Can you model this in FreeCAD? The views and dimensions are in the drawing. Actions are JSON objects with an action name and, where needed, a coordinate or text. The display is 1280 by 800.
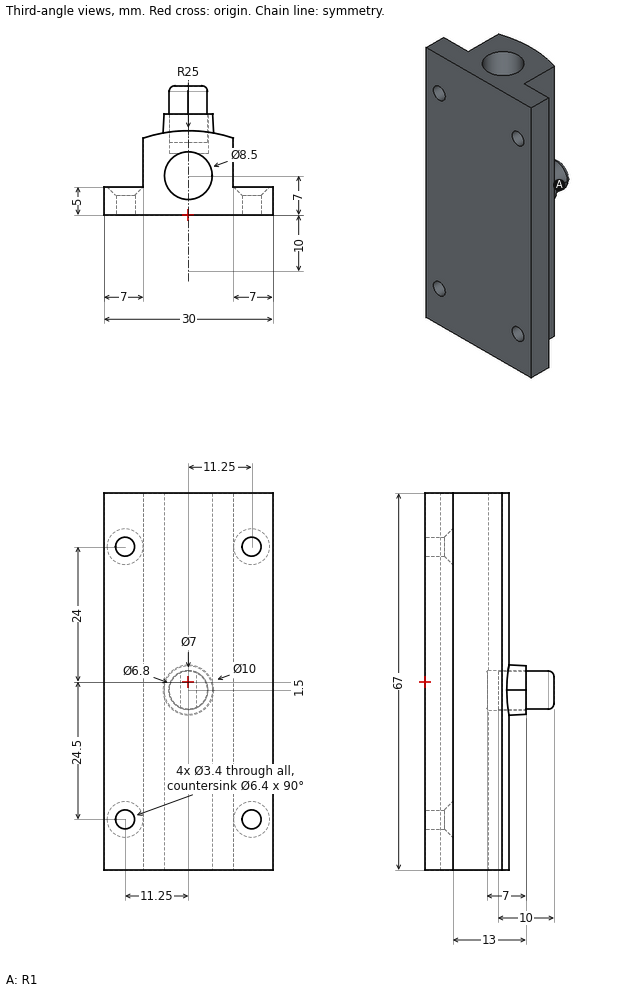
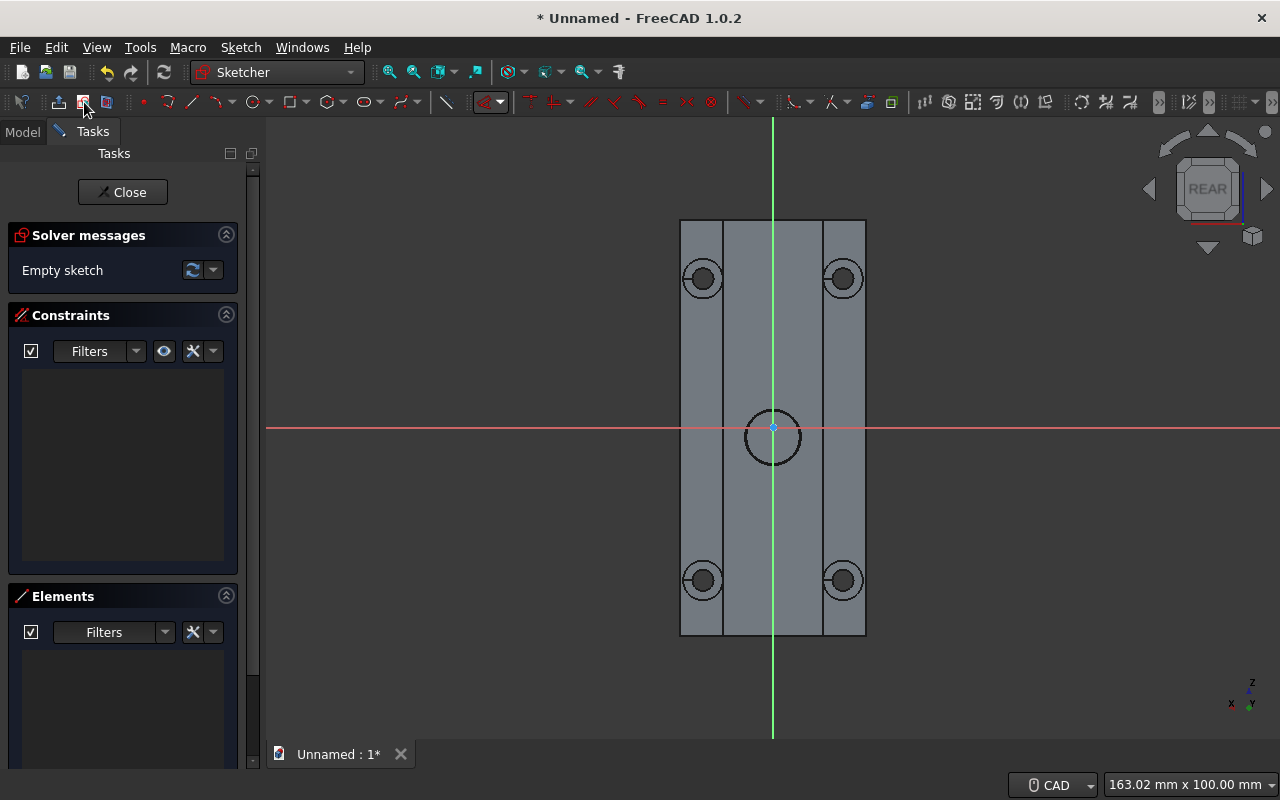
{"action": "scroll", "coordinate": [782, 438], "scroll_direction": "up", "scroll_amount": 11}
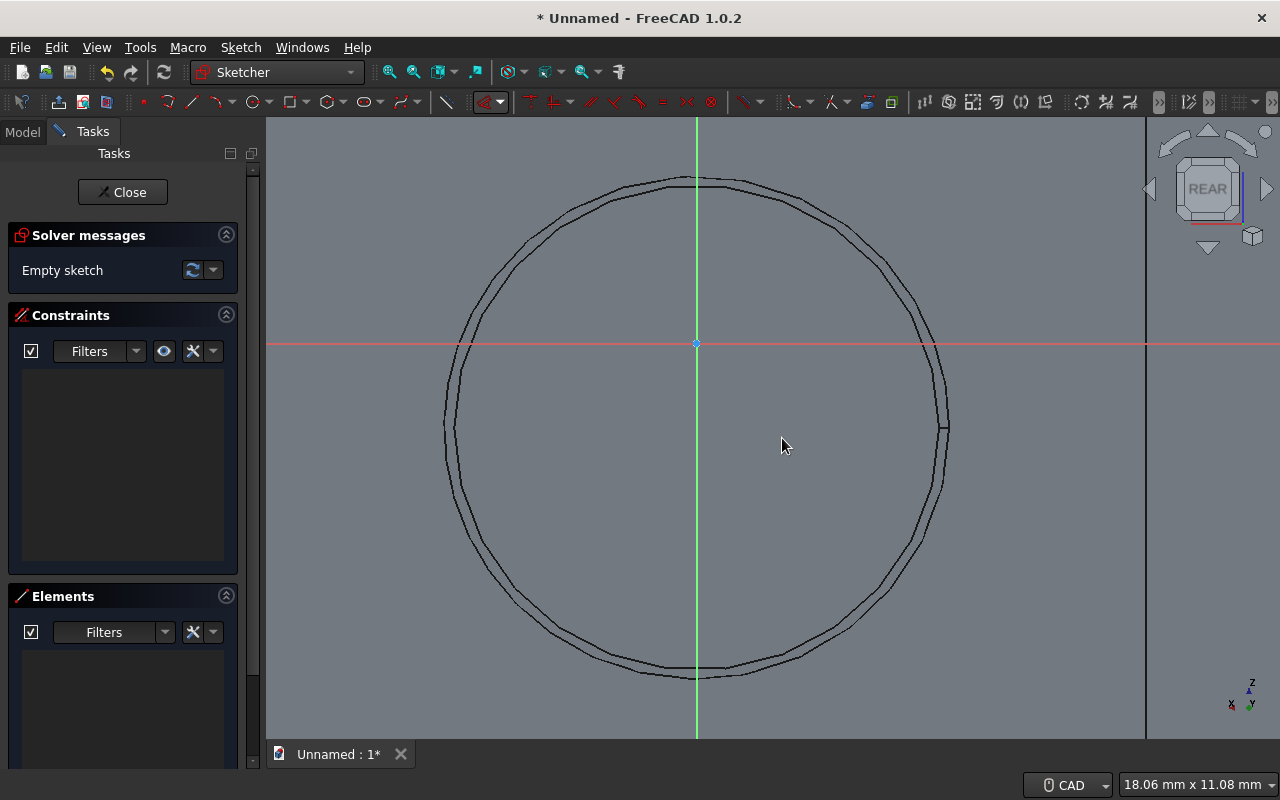
{"action": "key", "text": "g c"}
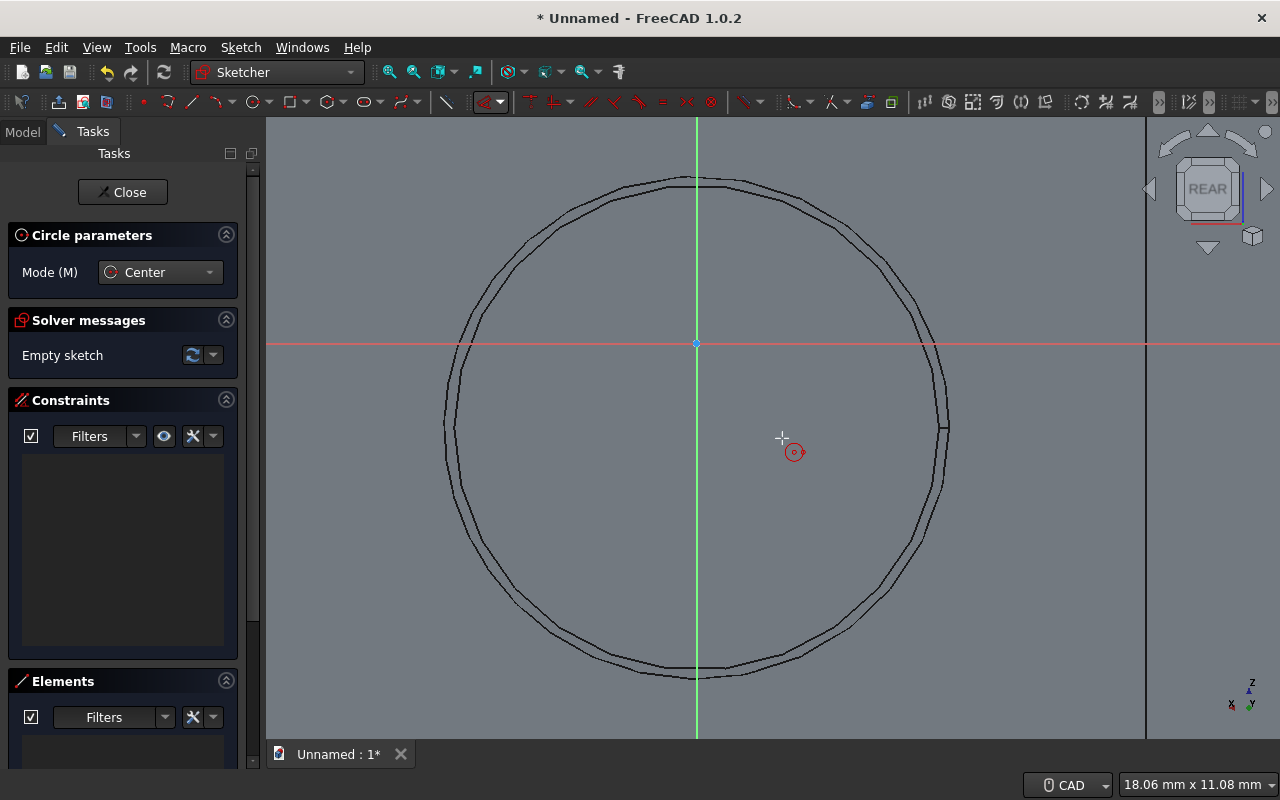
{"action": "left_click", "coordinate": [697, 428]}
{"action": "left_click", "coordinate": [836, 289]}
{"action": "key", "text": "Escape"}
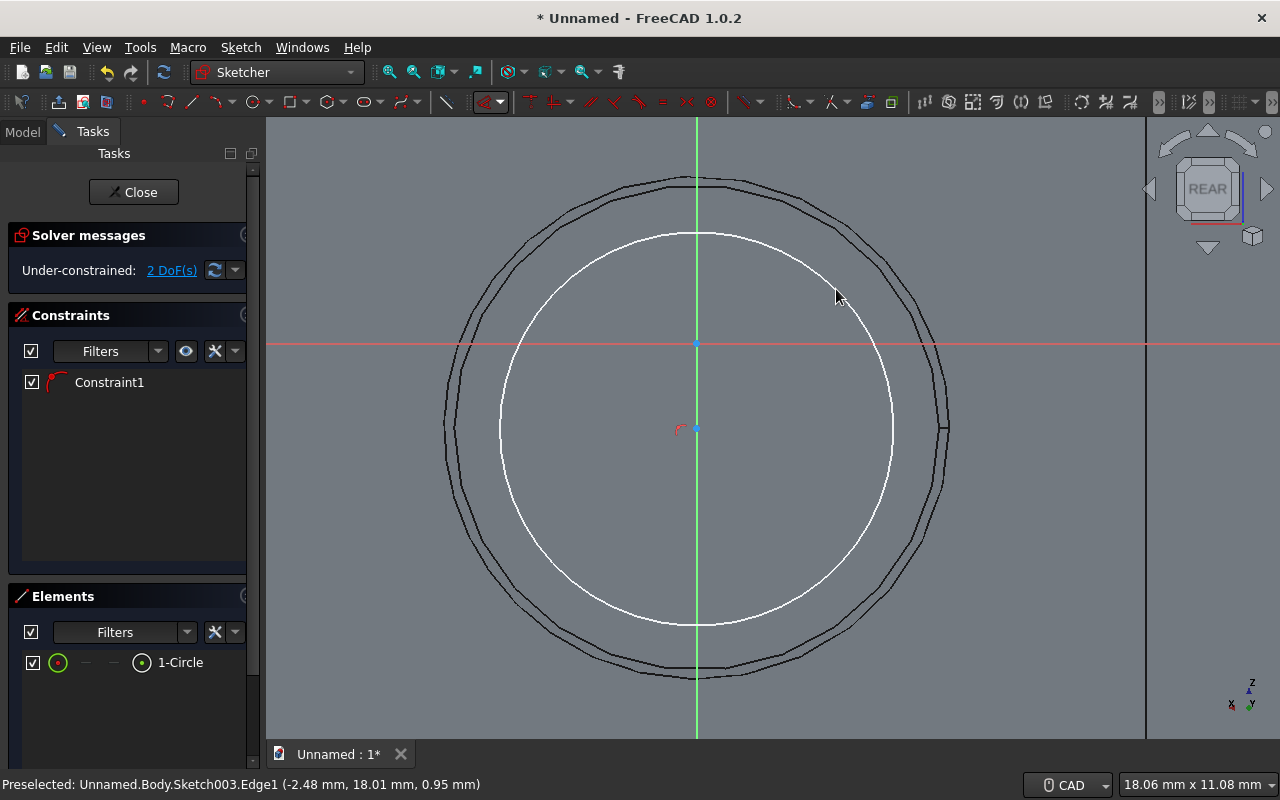
{"action": "left_click", "coordinate": [835, 289]}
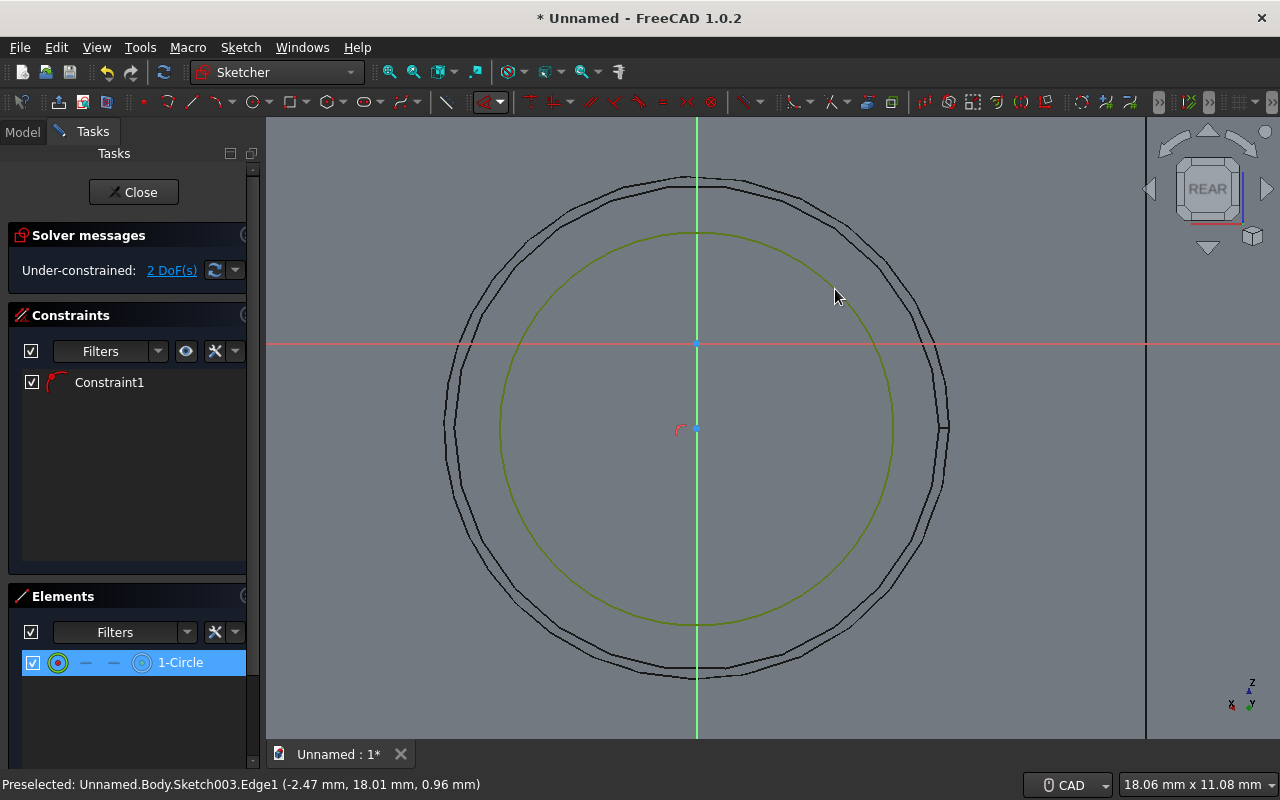
{"action": "key", "text": "k o"}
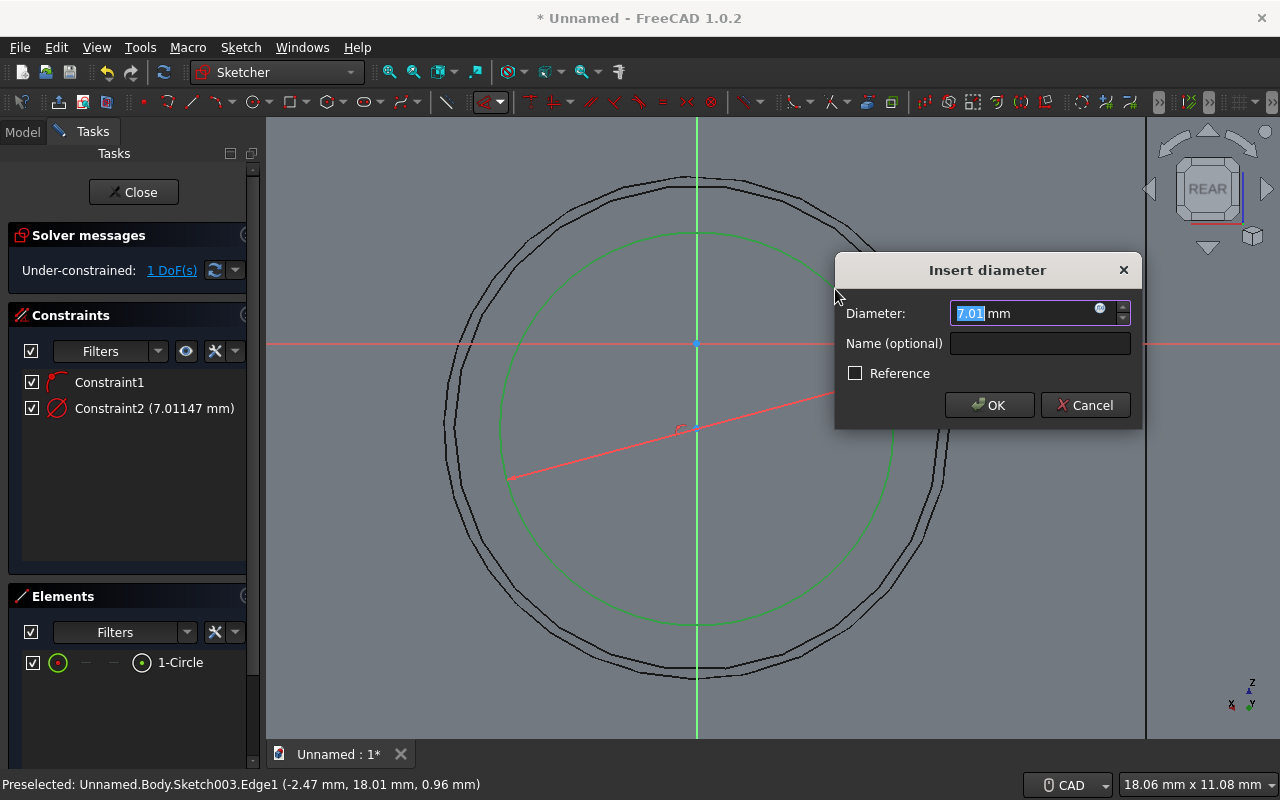
{"action": "type", "text": "7"}
{"action": "key", "text": "Return"}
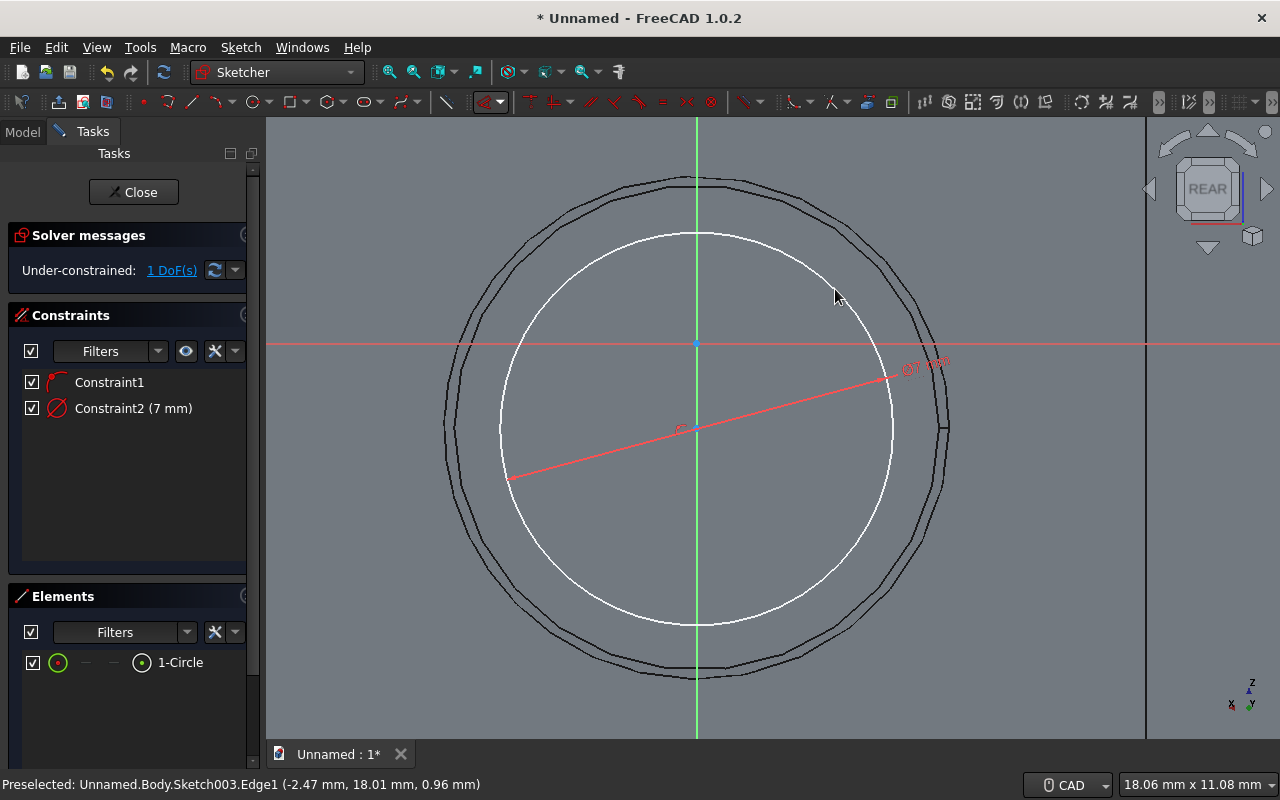
{"action": "left_click", "coordinate": [697, 429]}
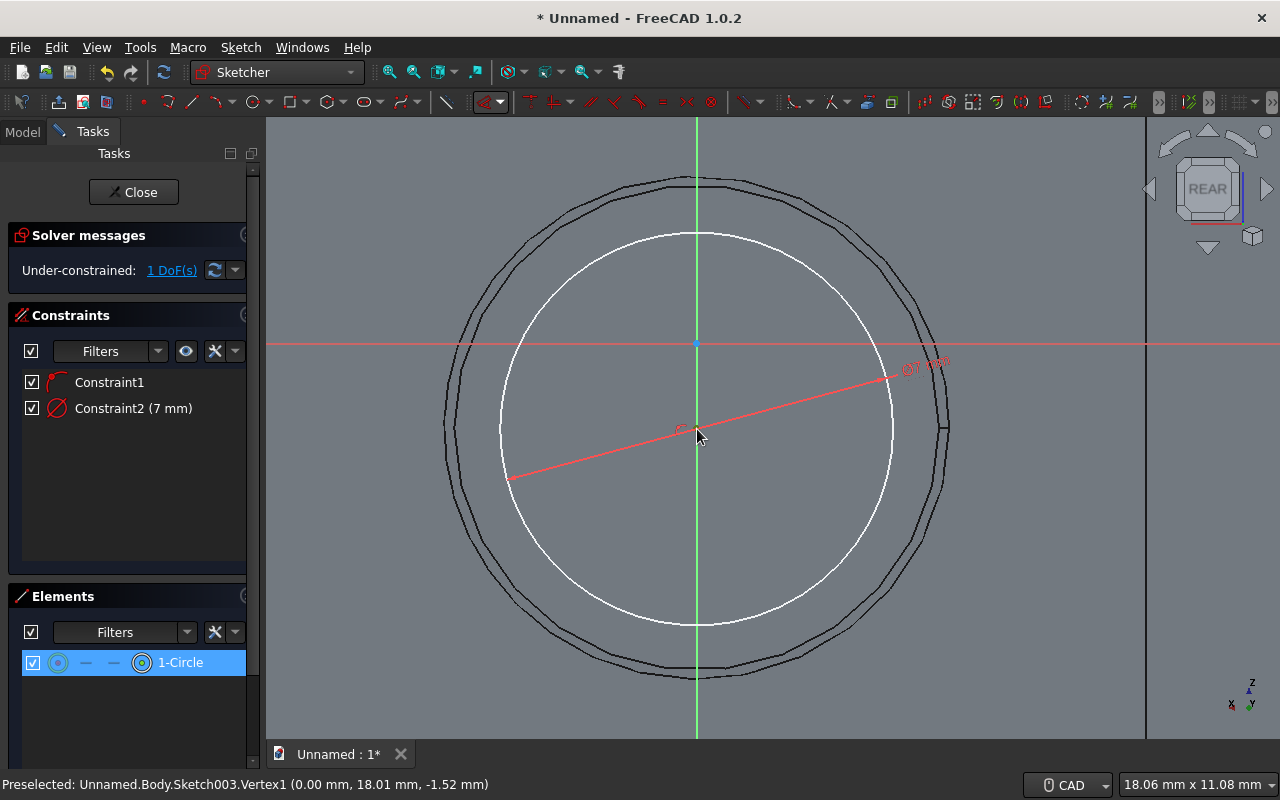
{"action": "key", "text": "i"}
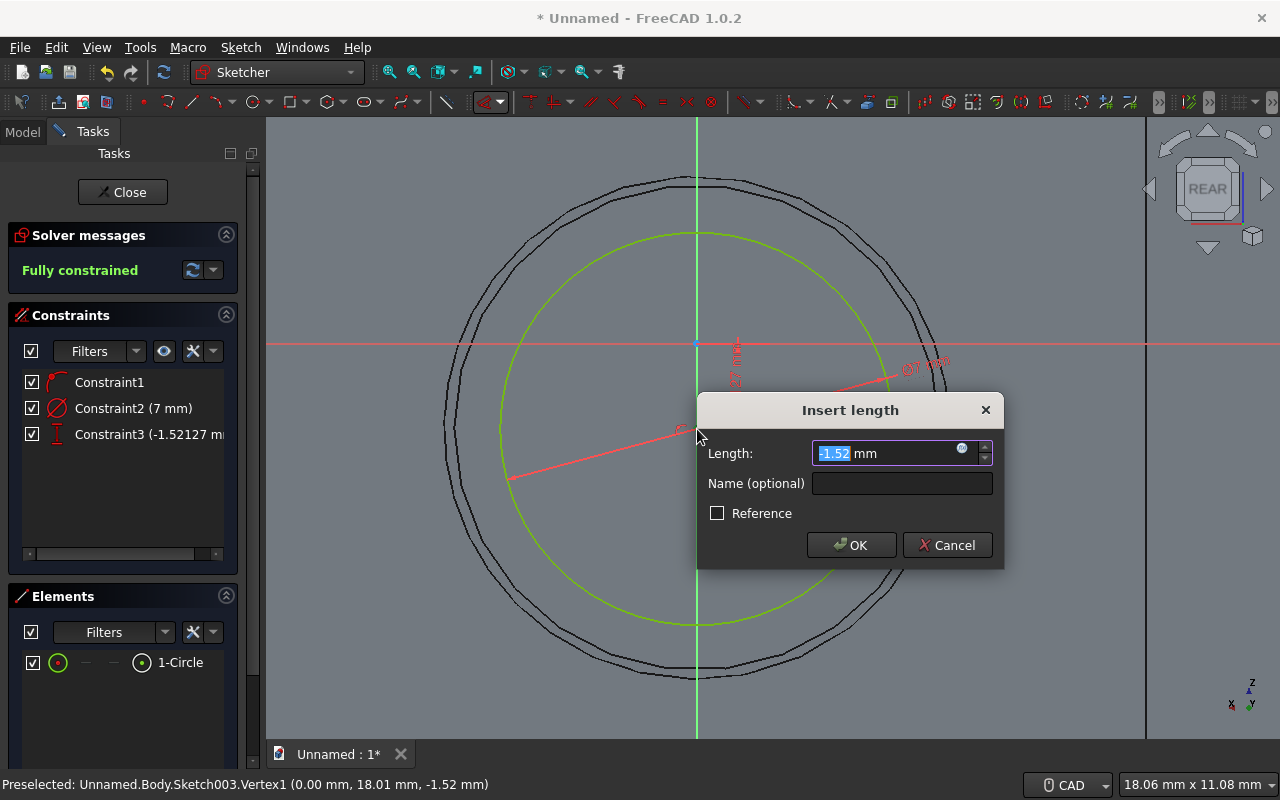
{"action": "type", "text": "-1.5"}
{"action": "key", "text": "Return"}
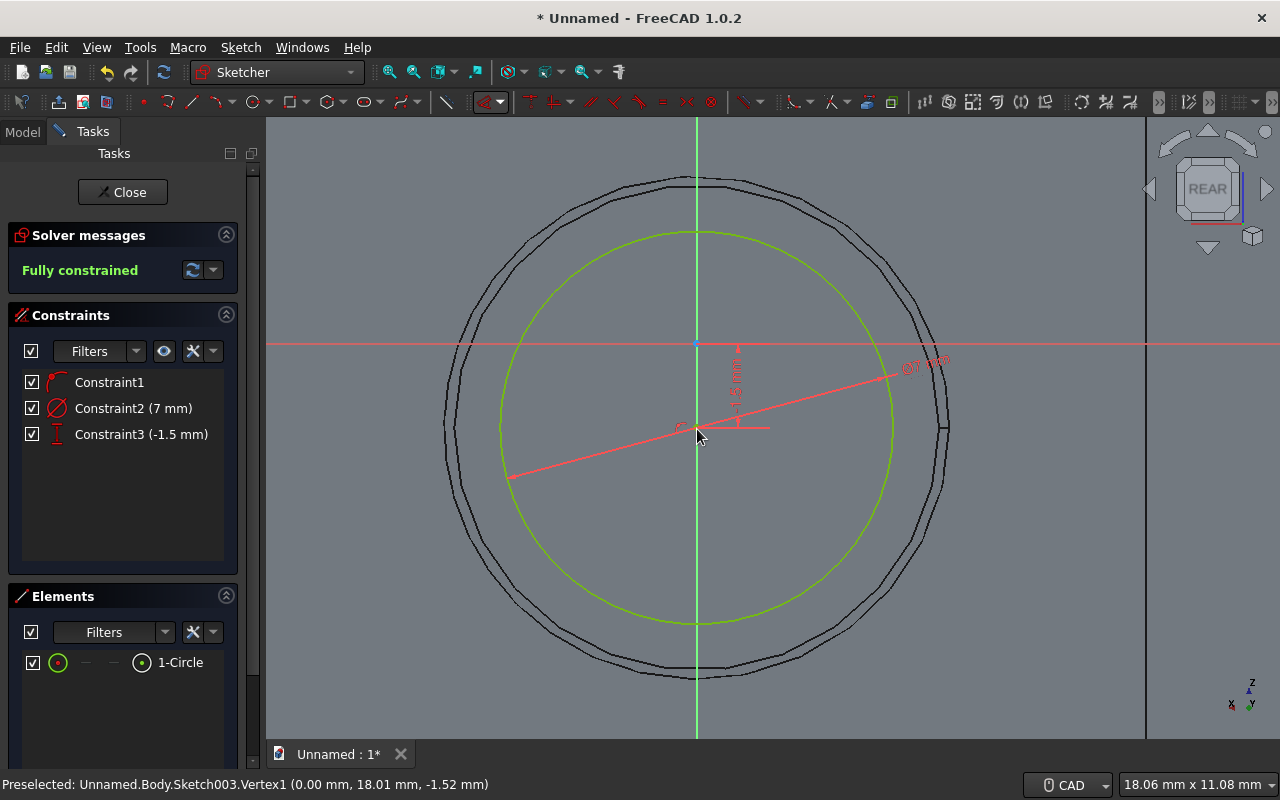
{"action": "left_click", "coordinate": [123, 192]}